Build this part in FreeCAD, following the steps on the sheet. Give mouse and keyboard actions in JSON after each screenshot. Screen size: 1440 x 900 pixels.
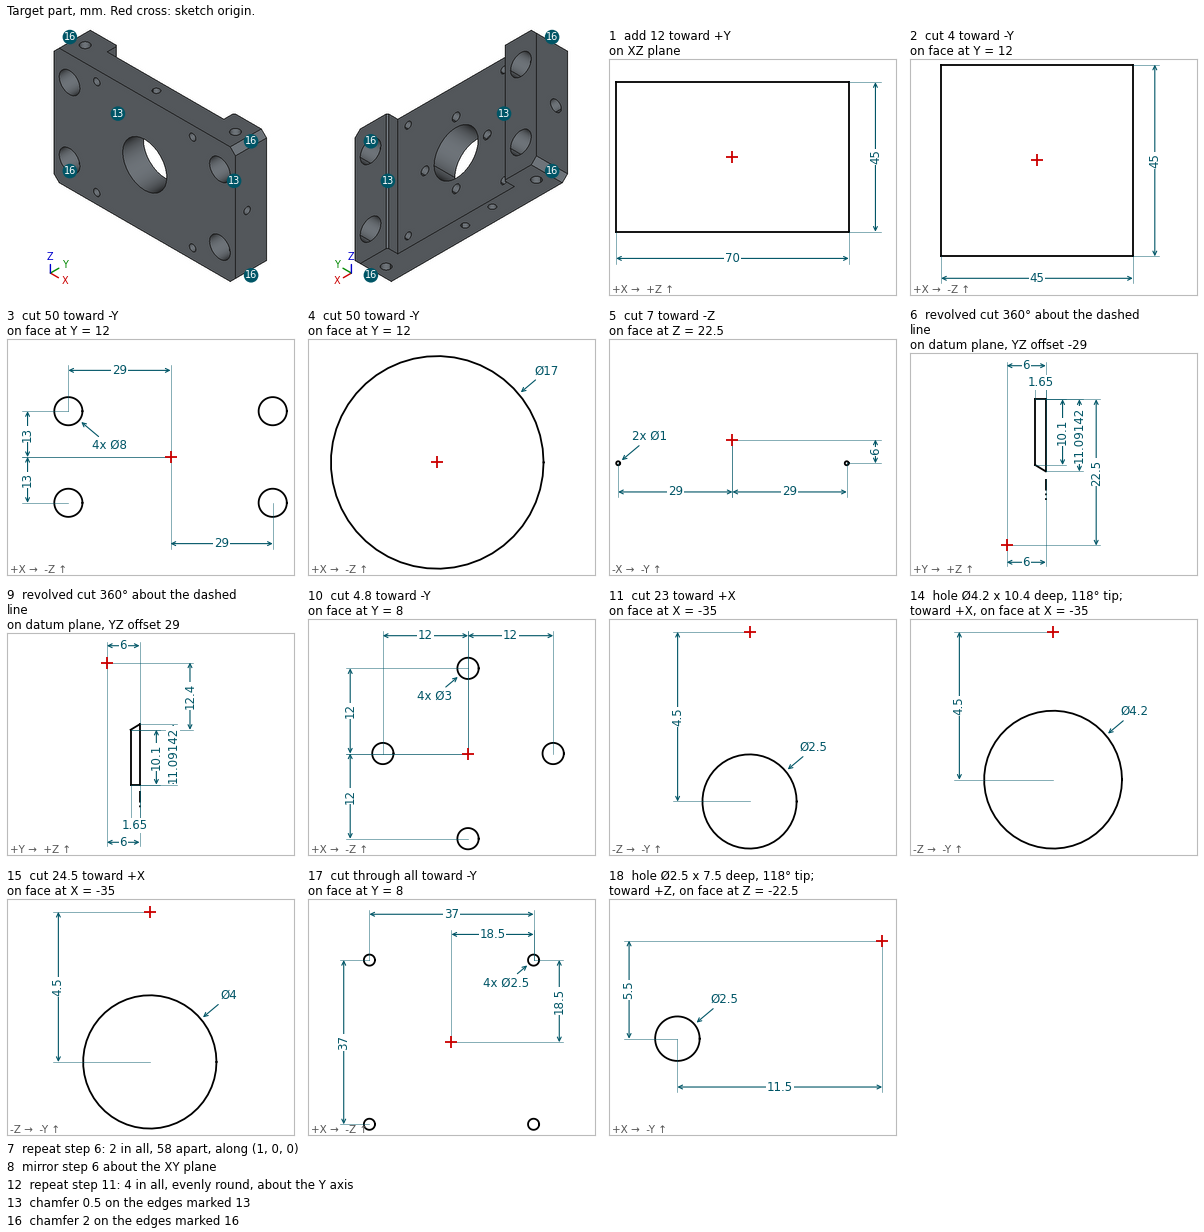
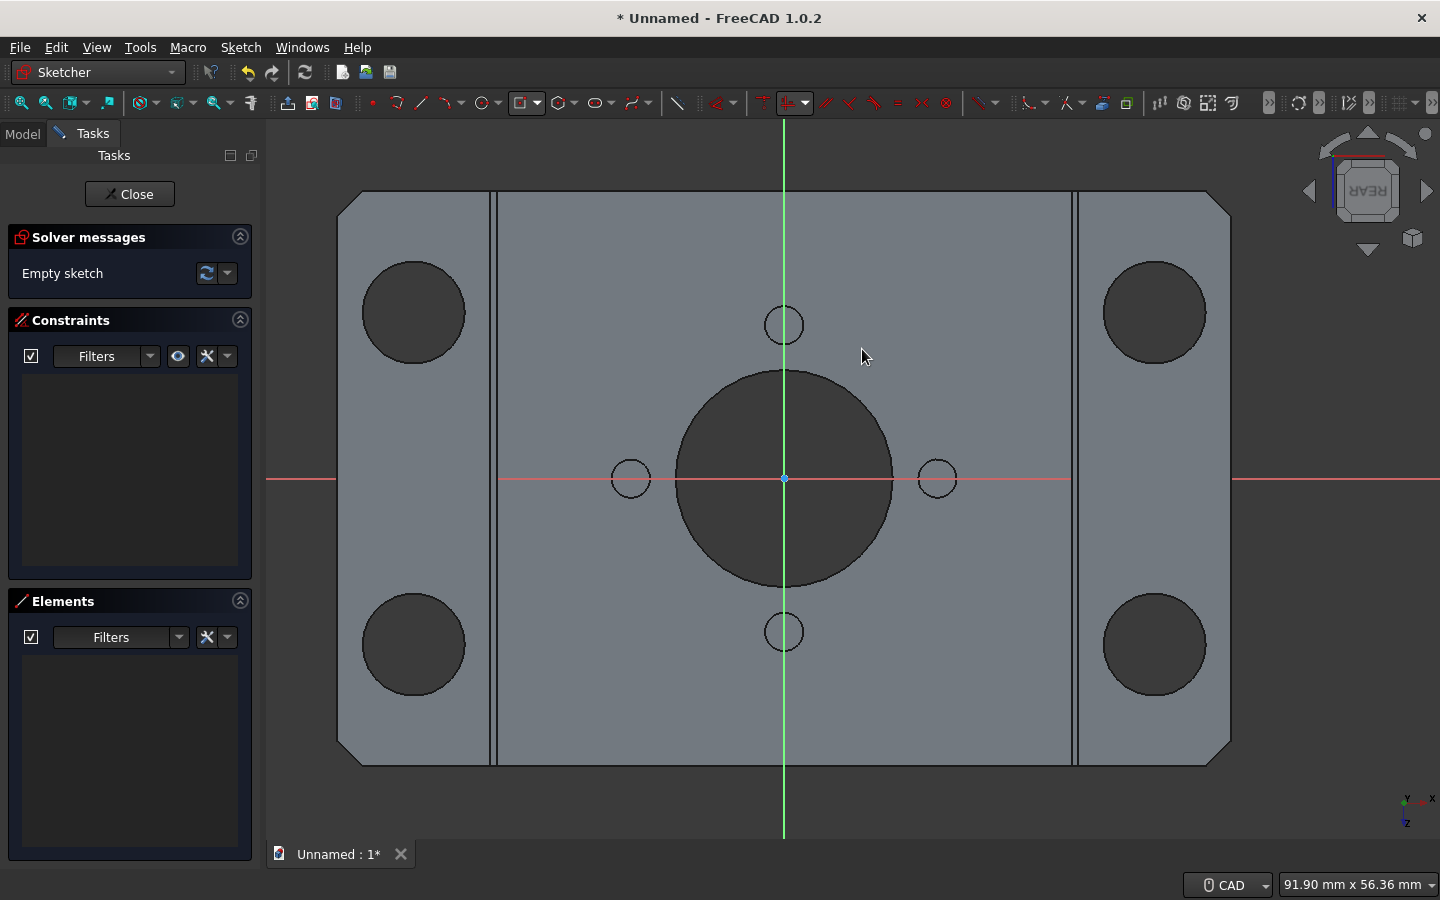
{"action": "left_click", "coordinate": [482, 104]}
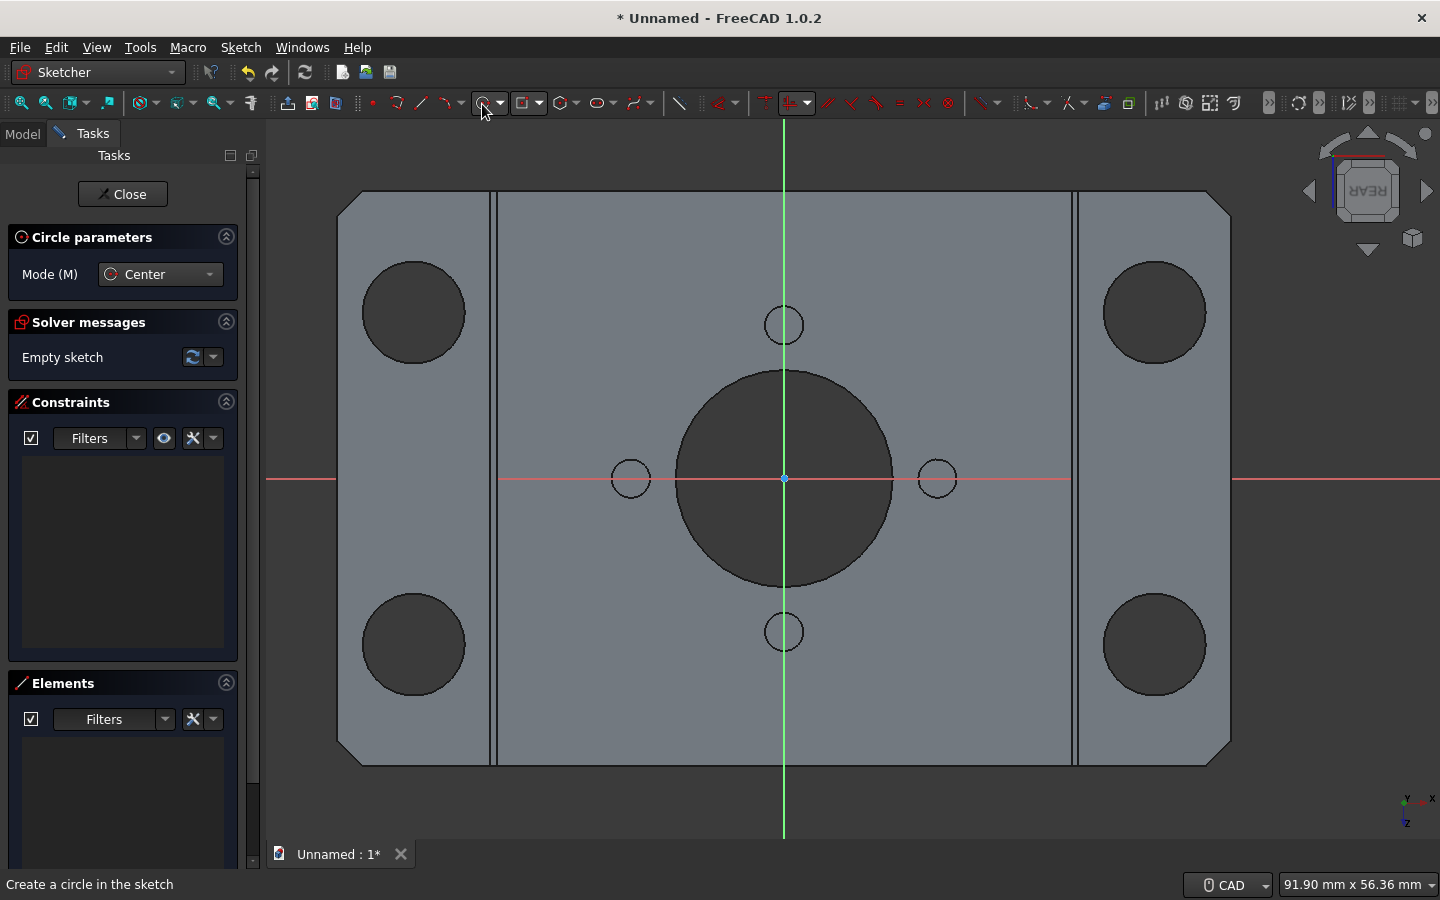
{"action": "scroll", "coordinate": [1020, 242], "scroll_direction": "up", "scroll_amount": 2}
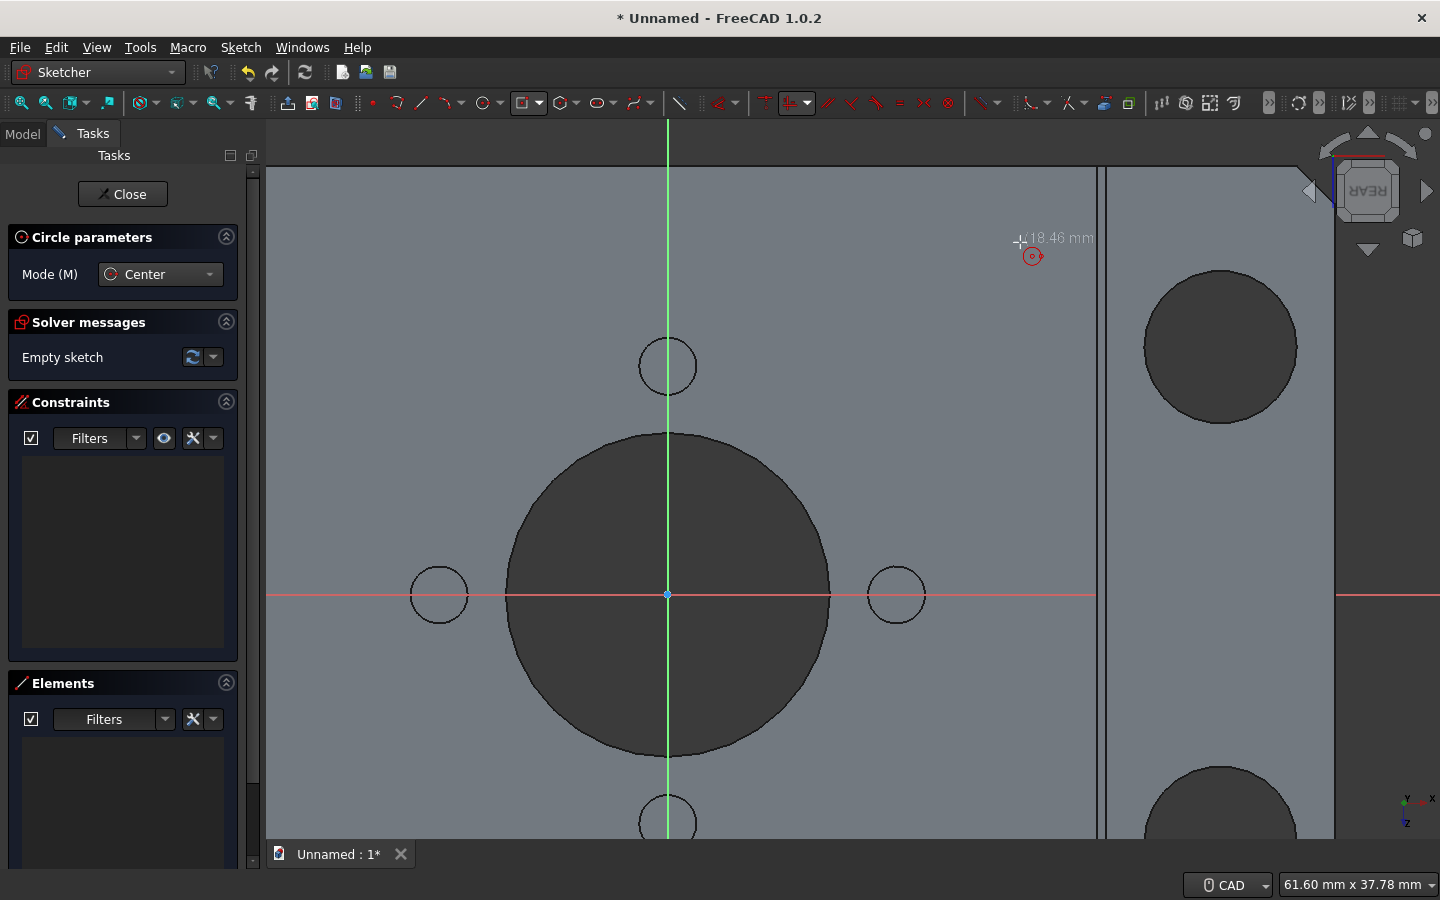
{"action": "left_click", "coordinate": [1020, 242]}
{"action": "mouse_move", "coordinate": [1037, 225]}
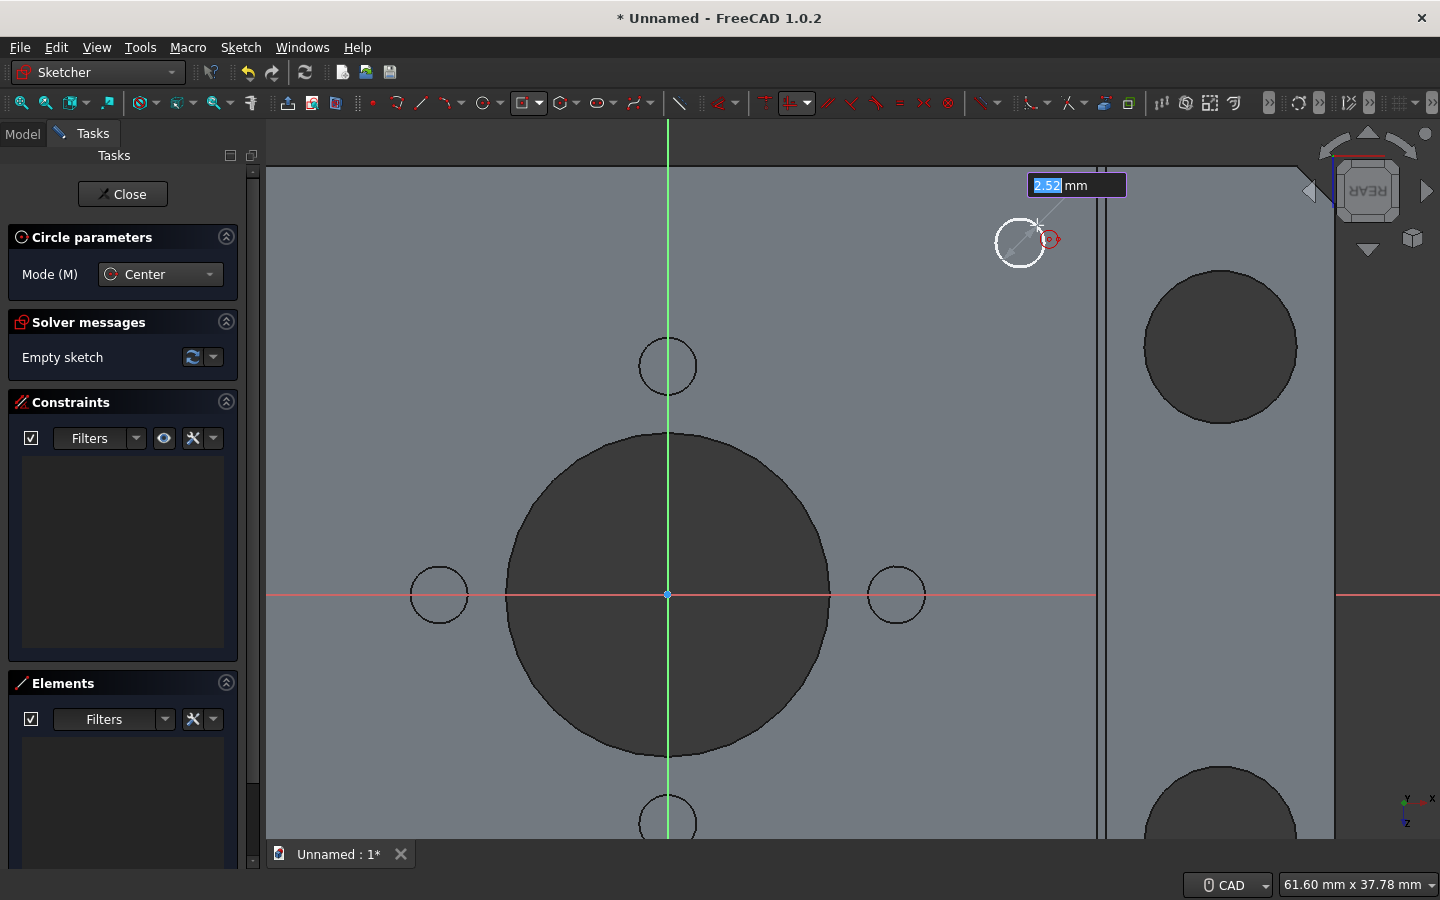
{"action": "type", "text": "2.5"}
{"action": "key", "text": "Return"}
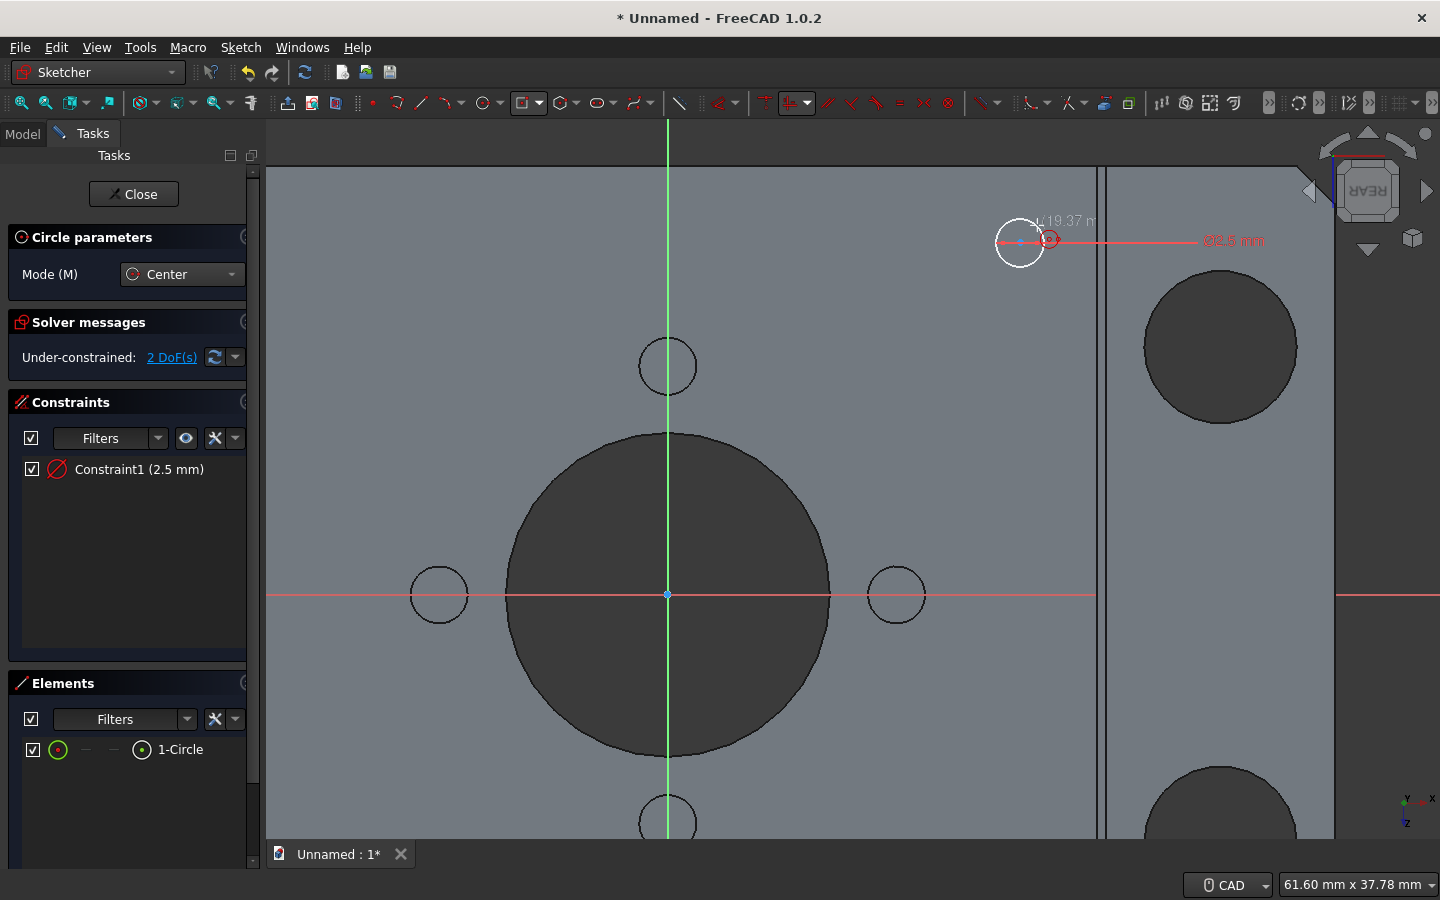
{"action": "left_click", "coordinate": [315, 242]}
{"action": "mouse_move", "coordinate": [332, 225]}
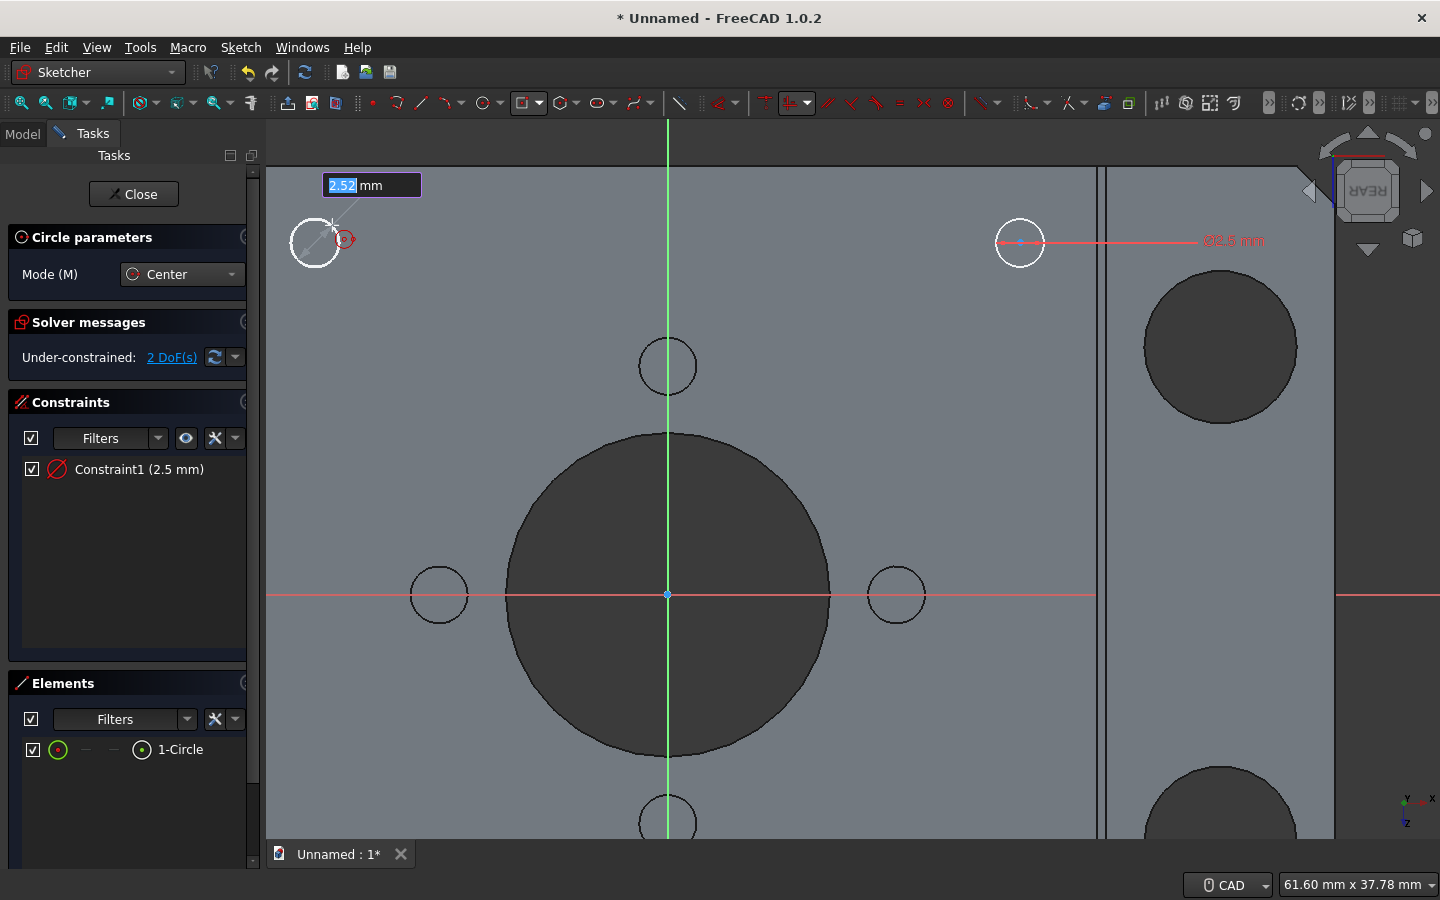
{"action": "type", "text": "2.5"}
{"action": "key", "text": "Return"}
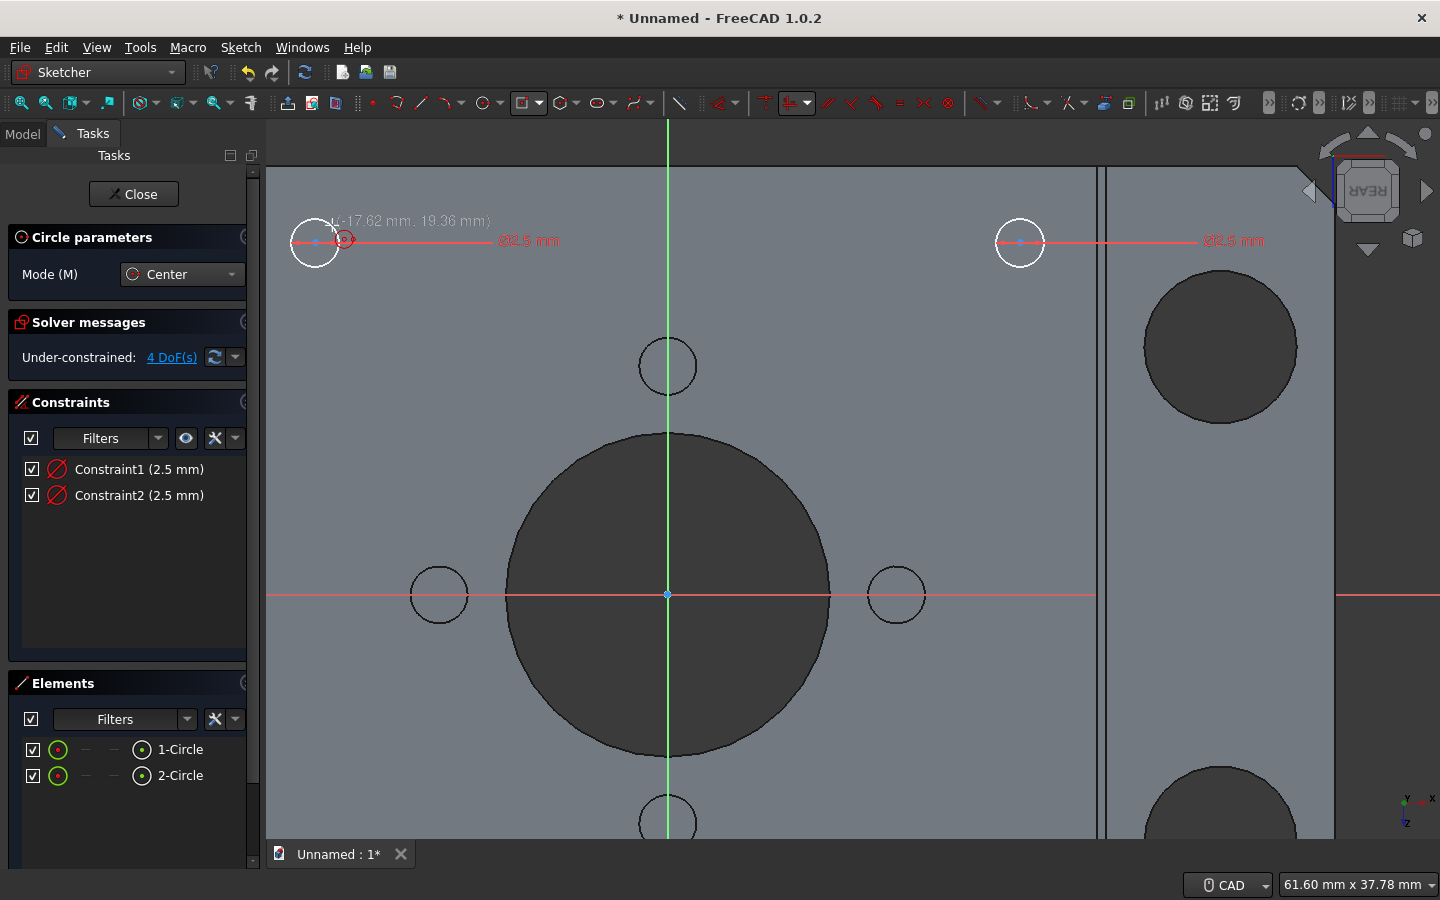
{"action": "scroll", "coordinate": [1022, 243], "scroll_direction": "down", "scroll_amount": 2}